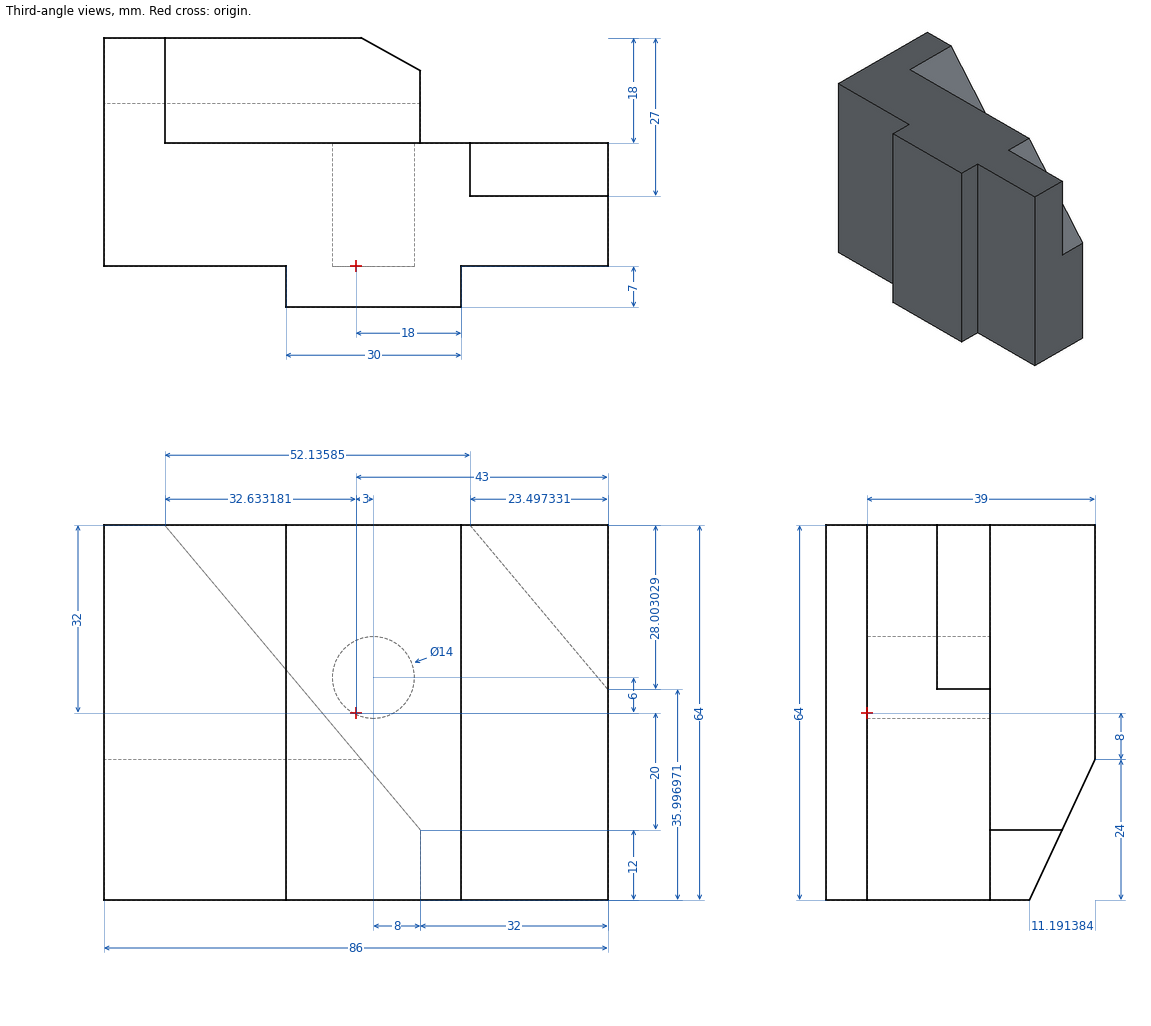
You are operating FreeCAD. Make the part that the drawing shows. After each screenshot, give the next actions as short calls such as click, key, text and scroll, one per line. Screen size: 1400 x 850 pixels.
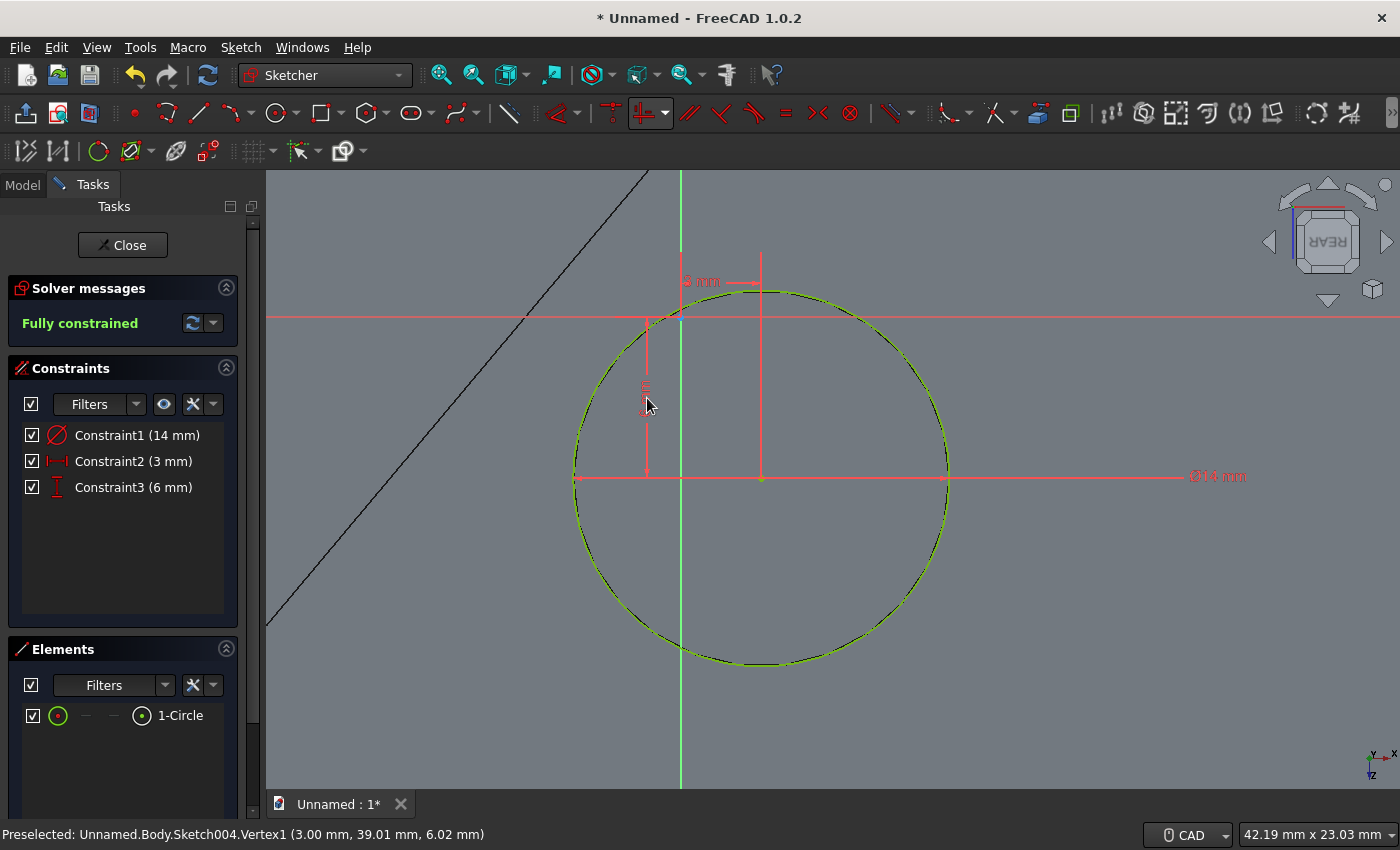
click(123, 245)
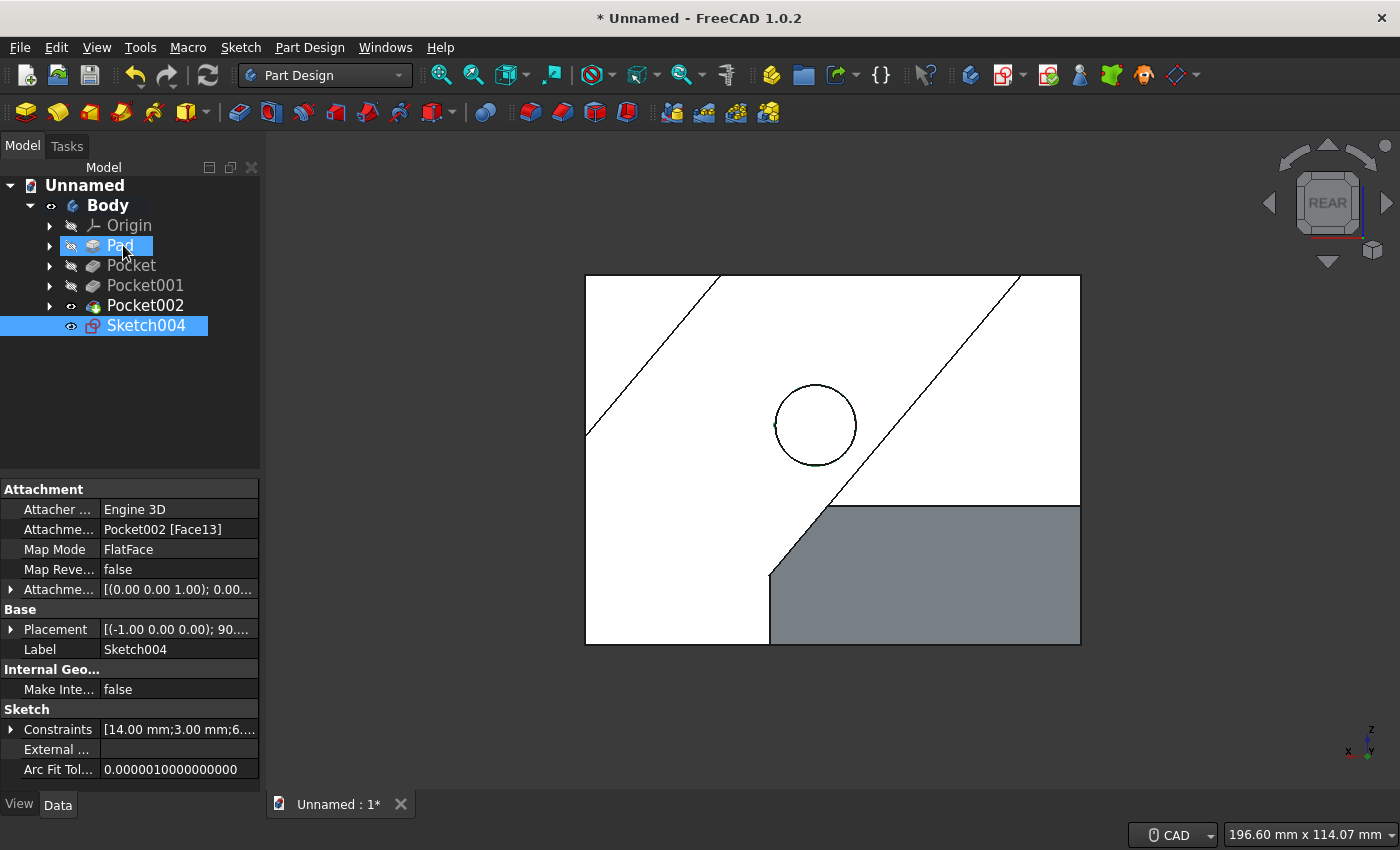
click(240, 112)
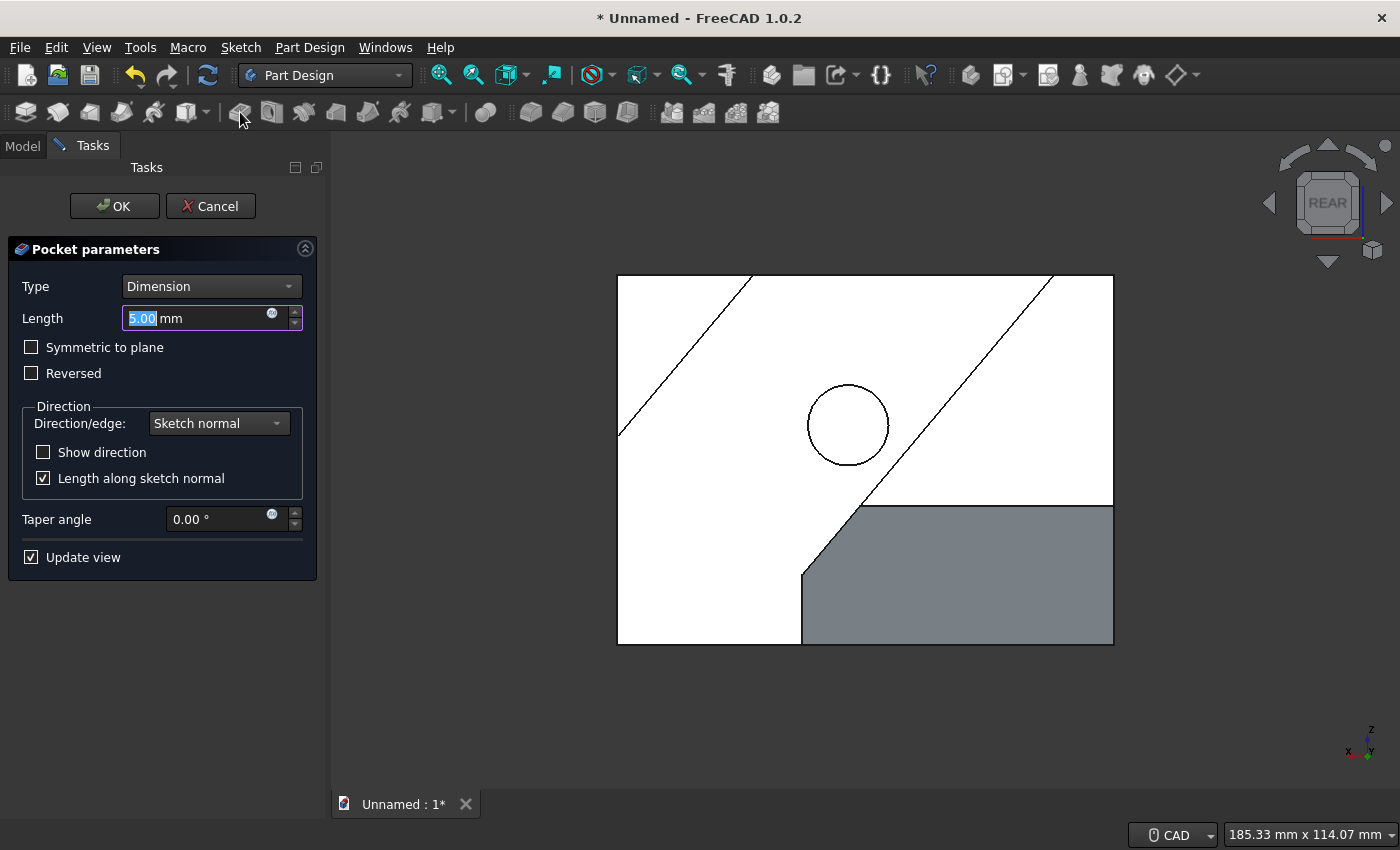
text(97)
key(Tab)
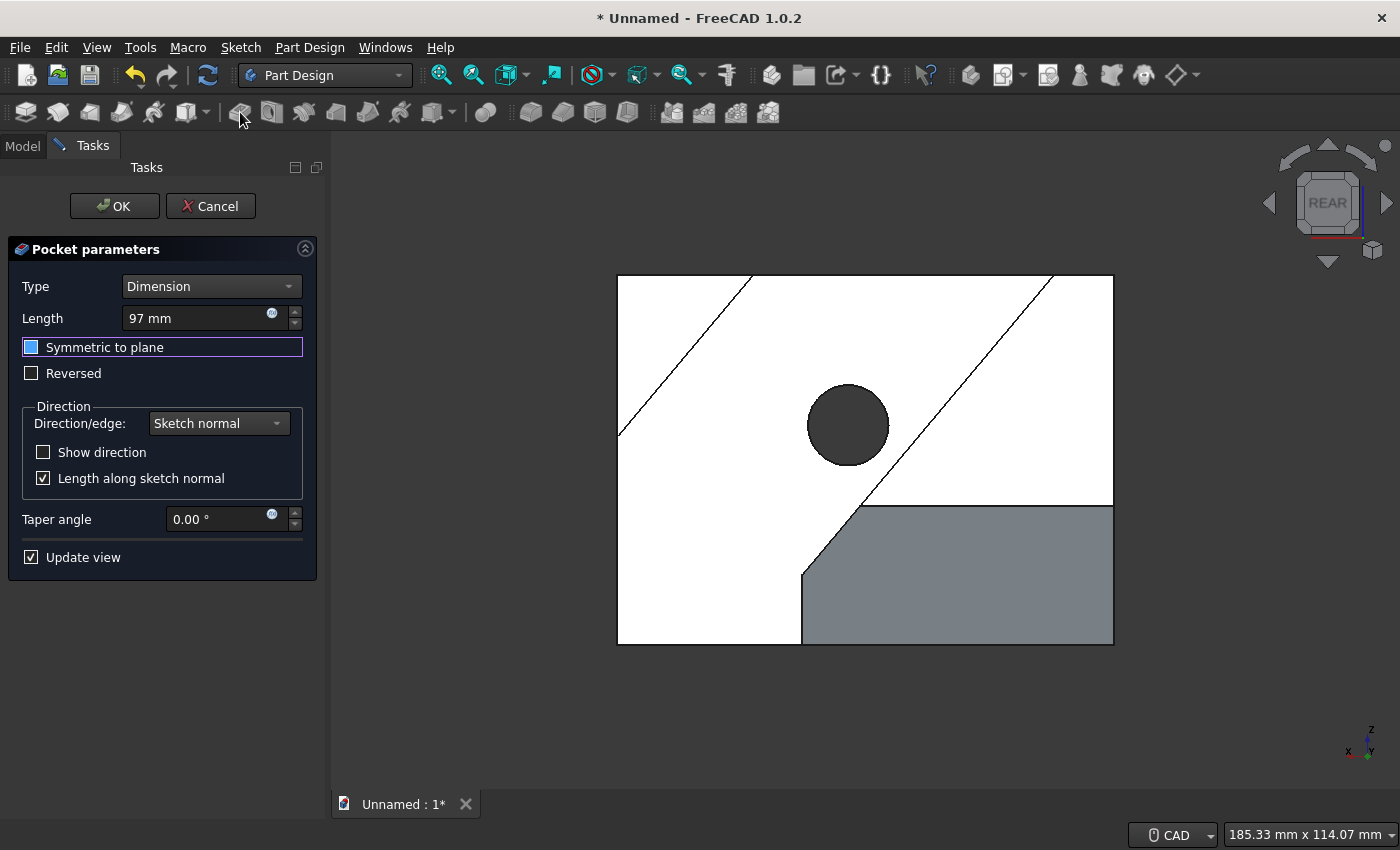
click(115, 206)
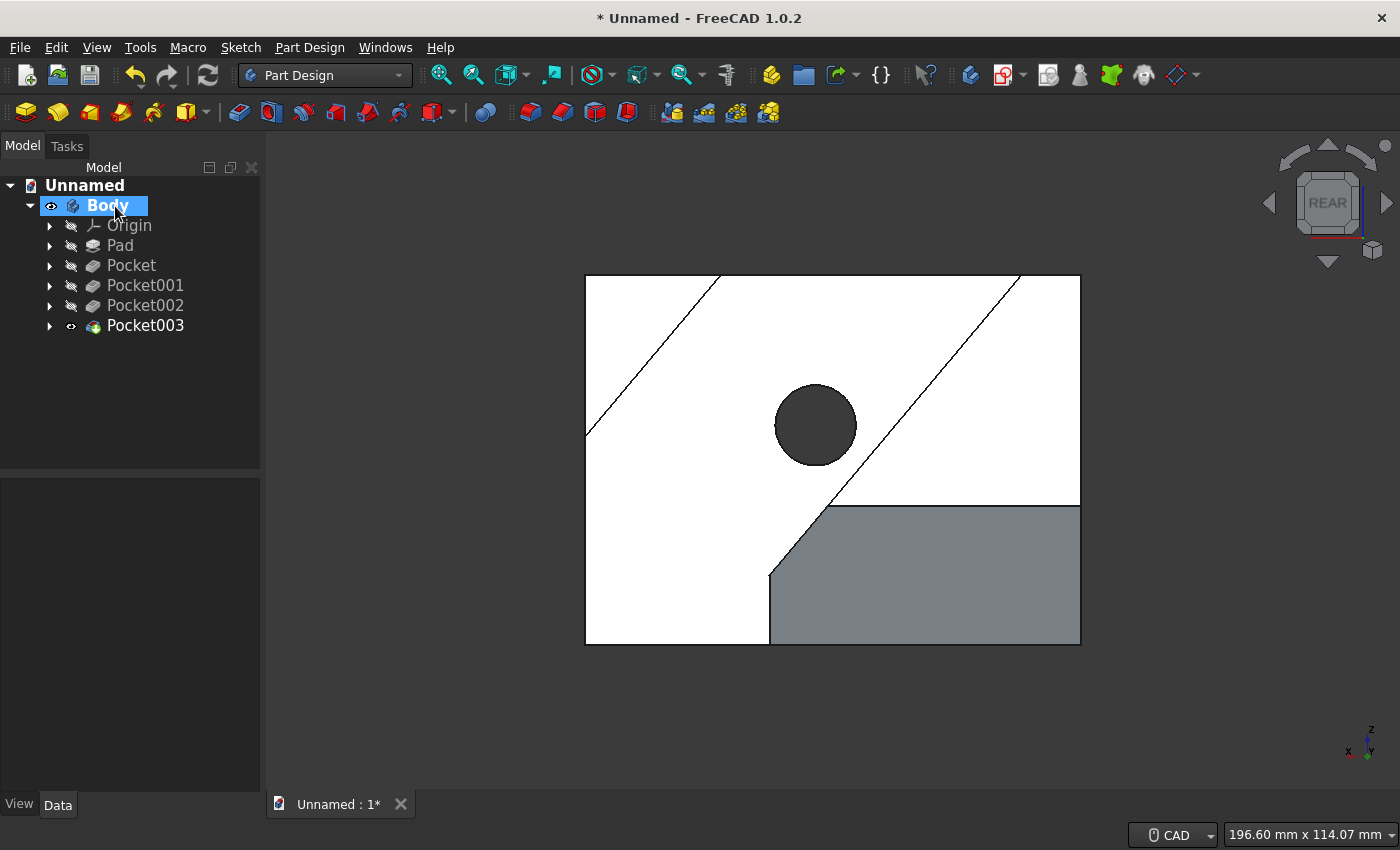
key(0)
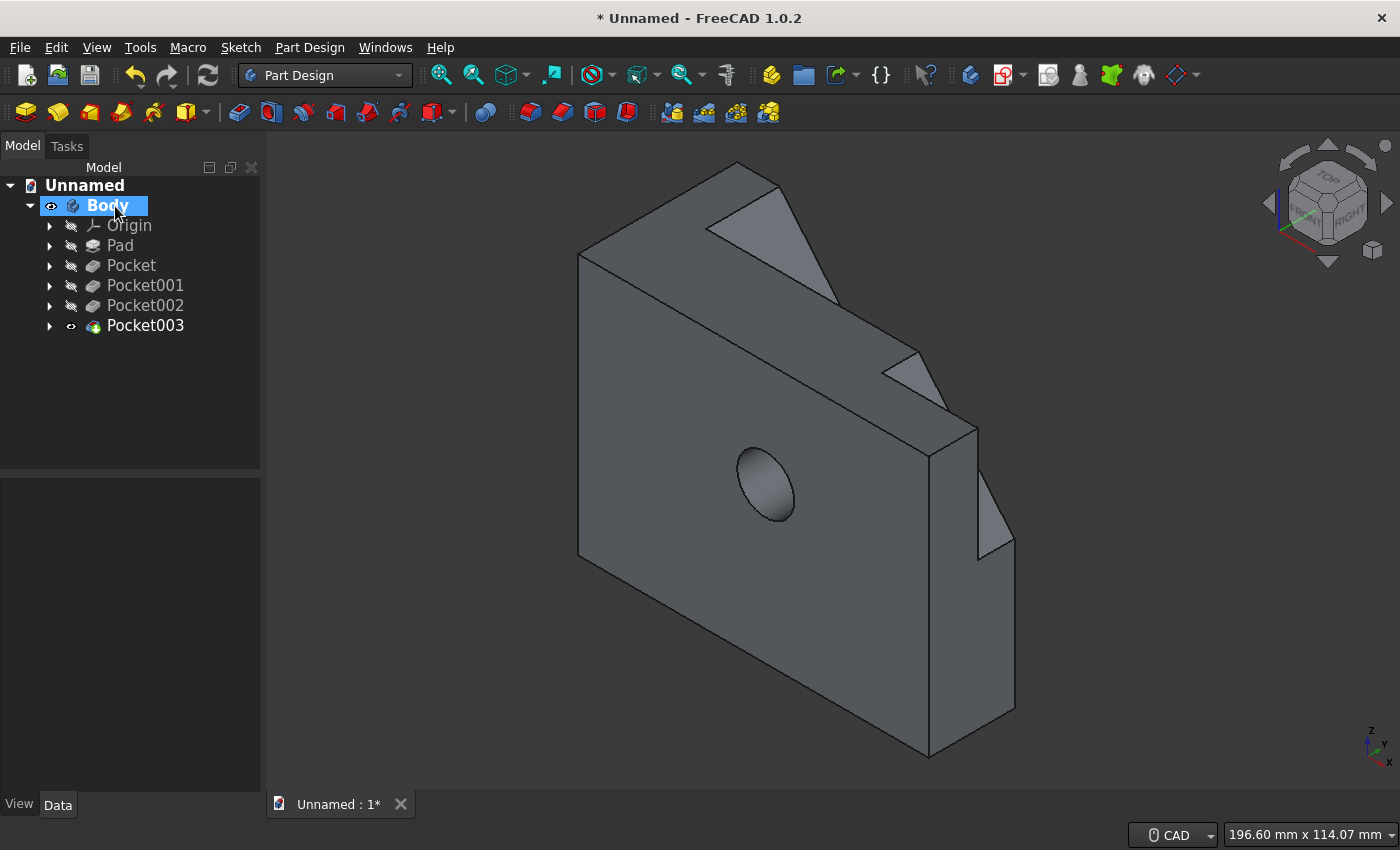
click(788, 335)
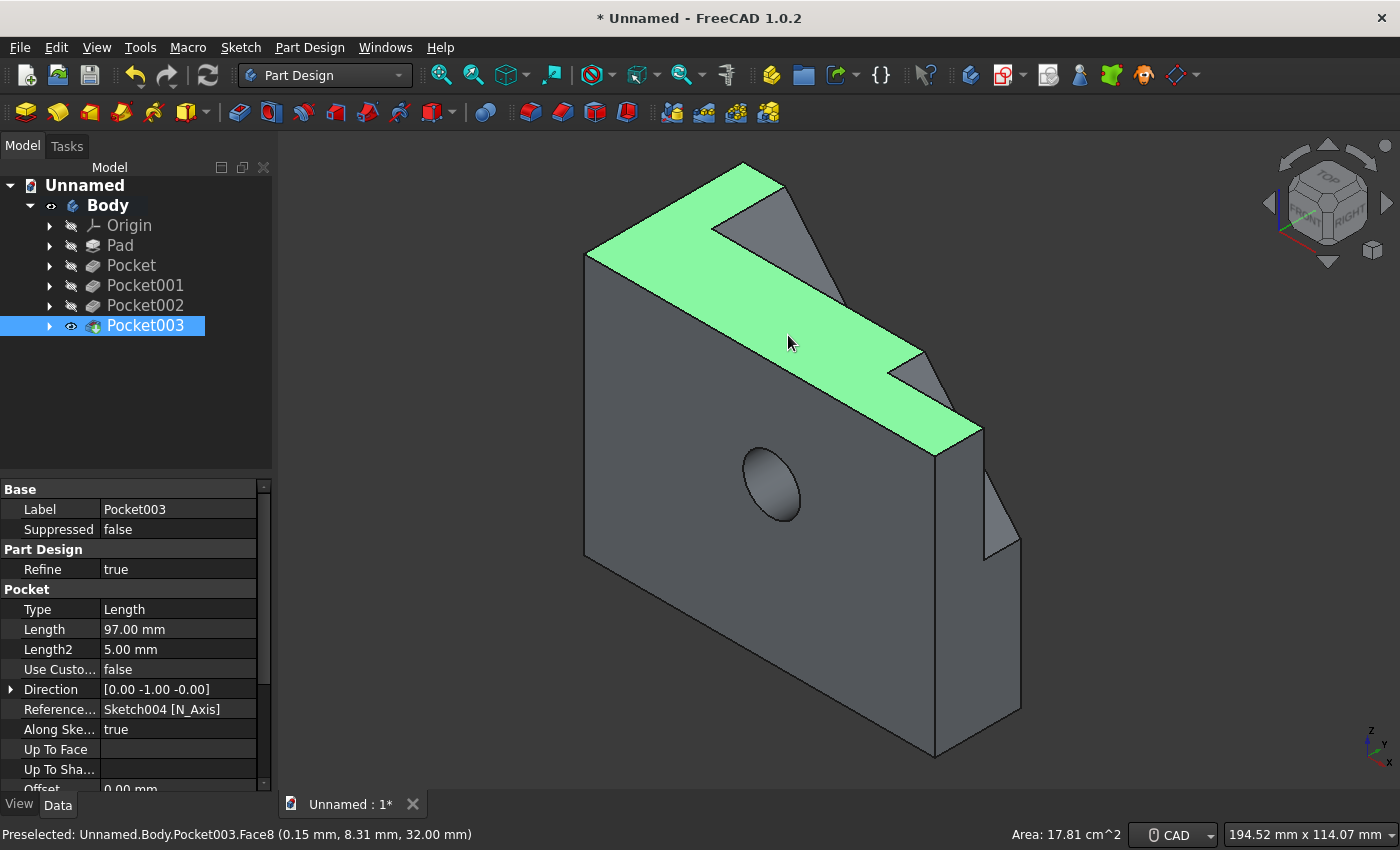
click(1004, 76)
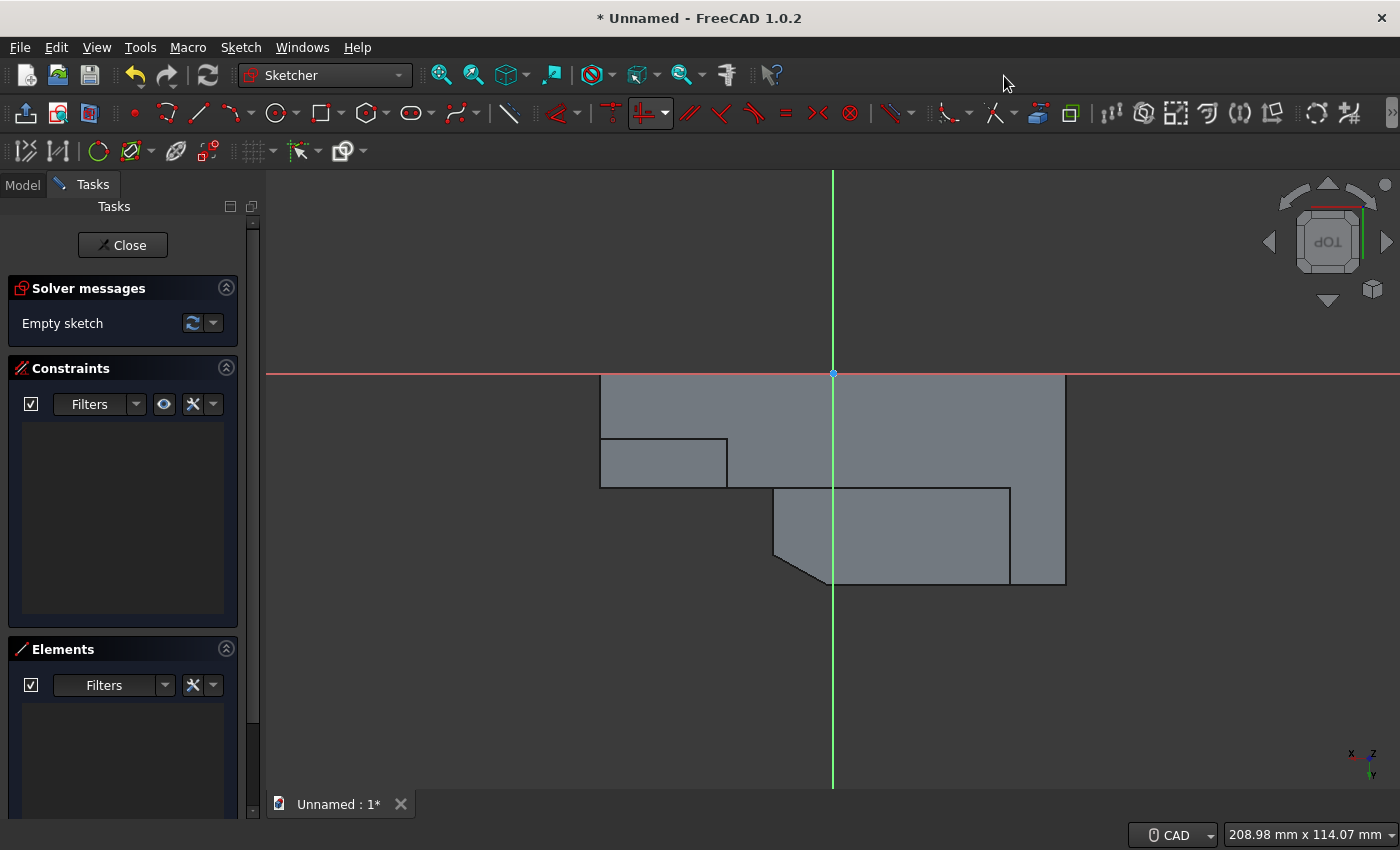
scroll(834, 314, up, 7)